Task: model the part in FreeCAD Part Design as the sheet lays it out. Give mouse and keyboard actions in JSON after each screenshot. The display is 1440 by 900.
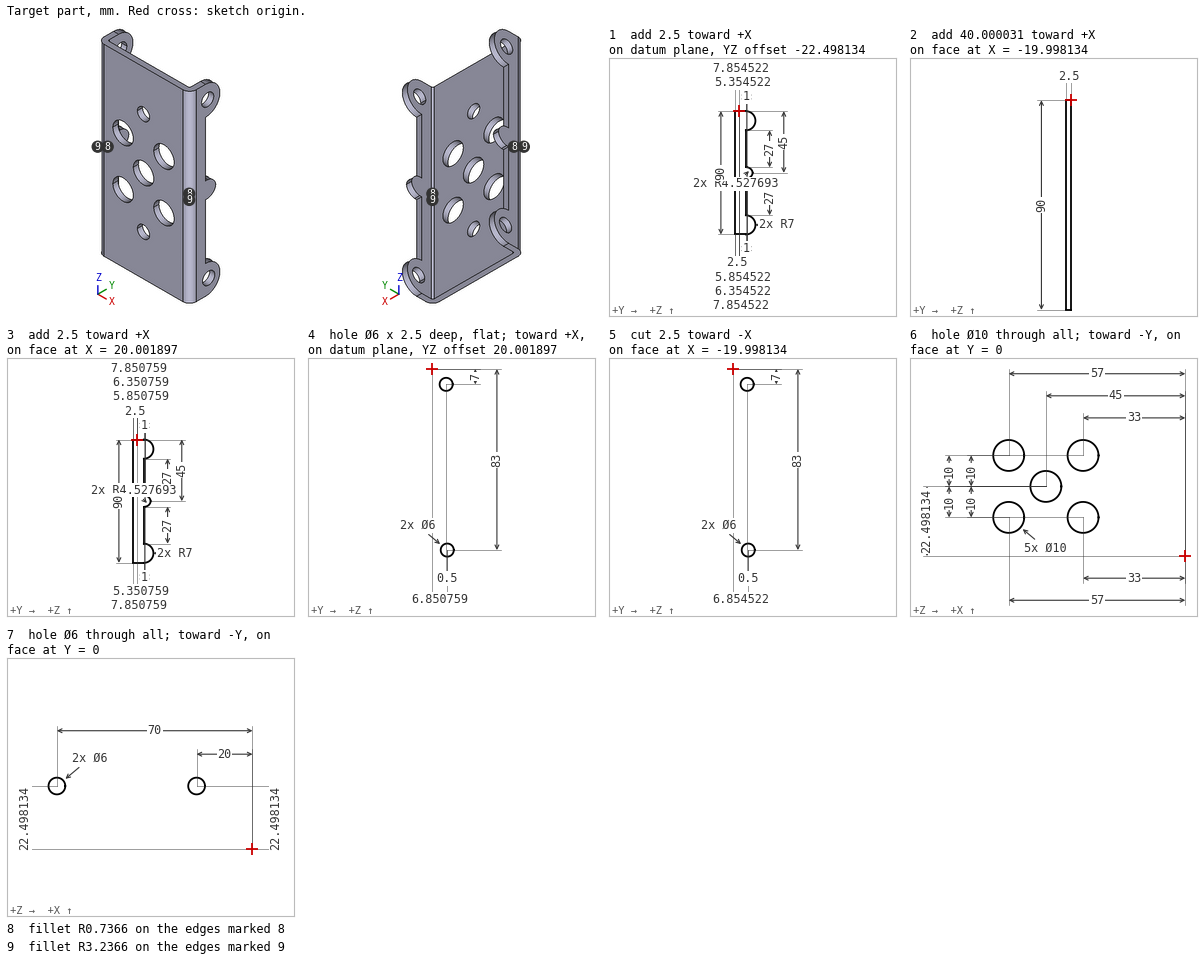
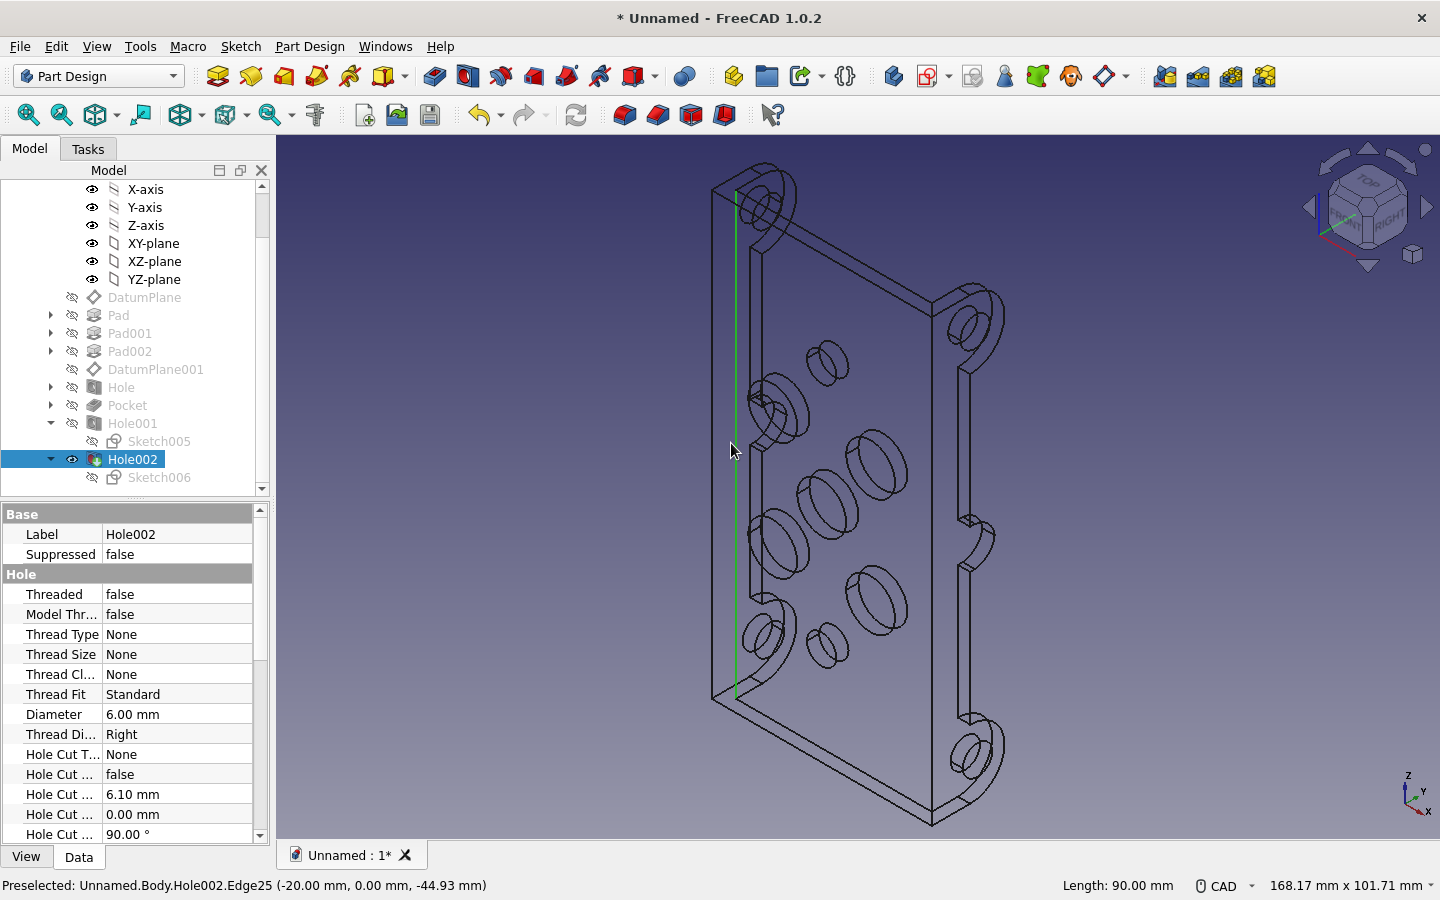
{"action": "scroll", "coordinate": [932, 556], "scroll_direction": "up", "scroll_amount": 6}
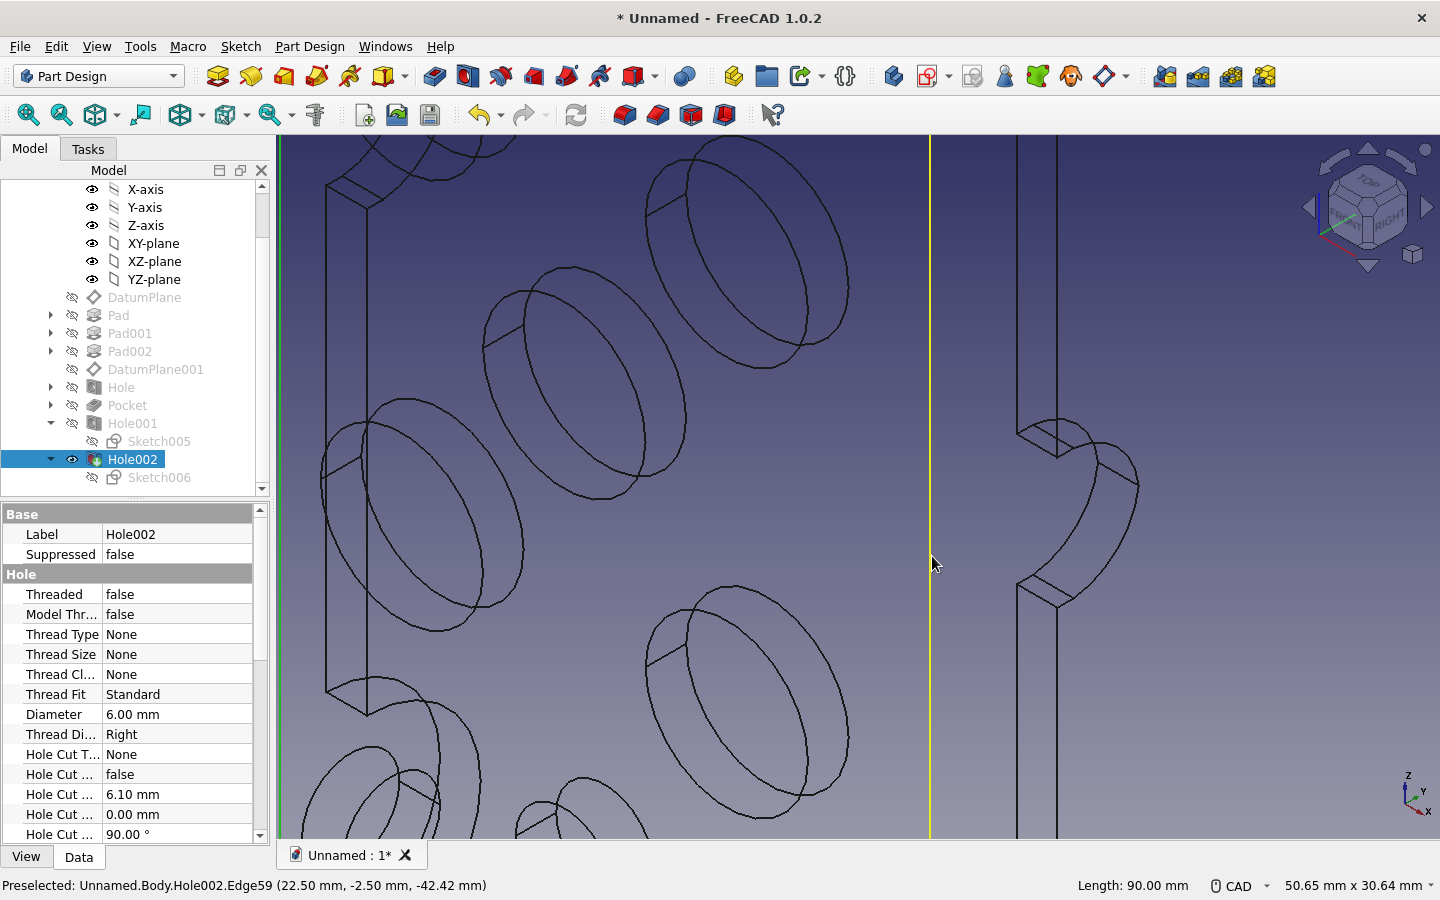
{"action": "left_click", "coordinate": [29, 116]}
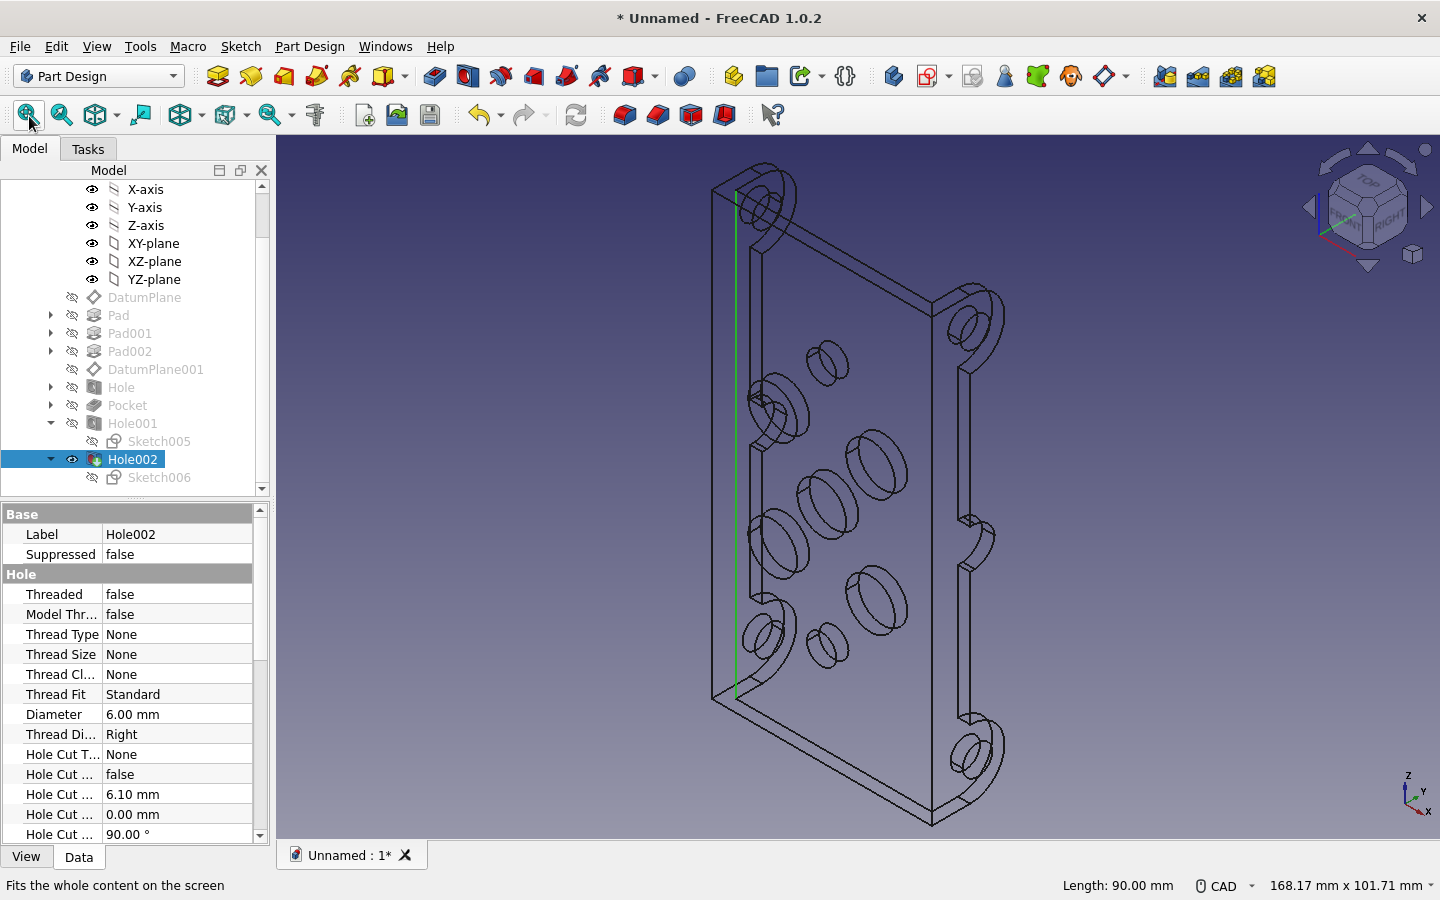
{"action": "key", "text": "2"}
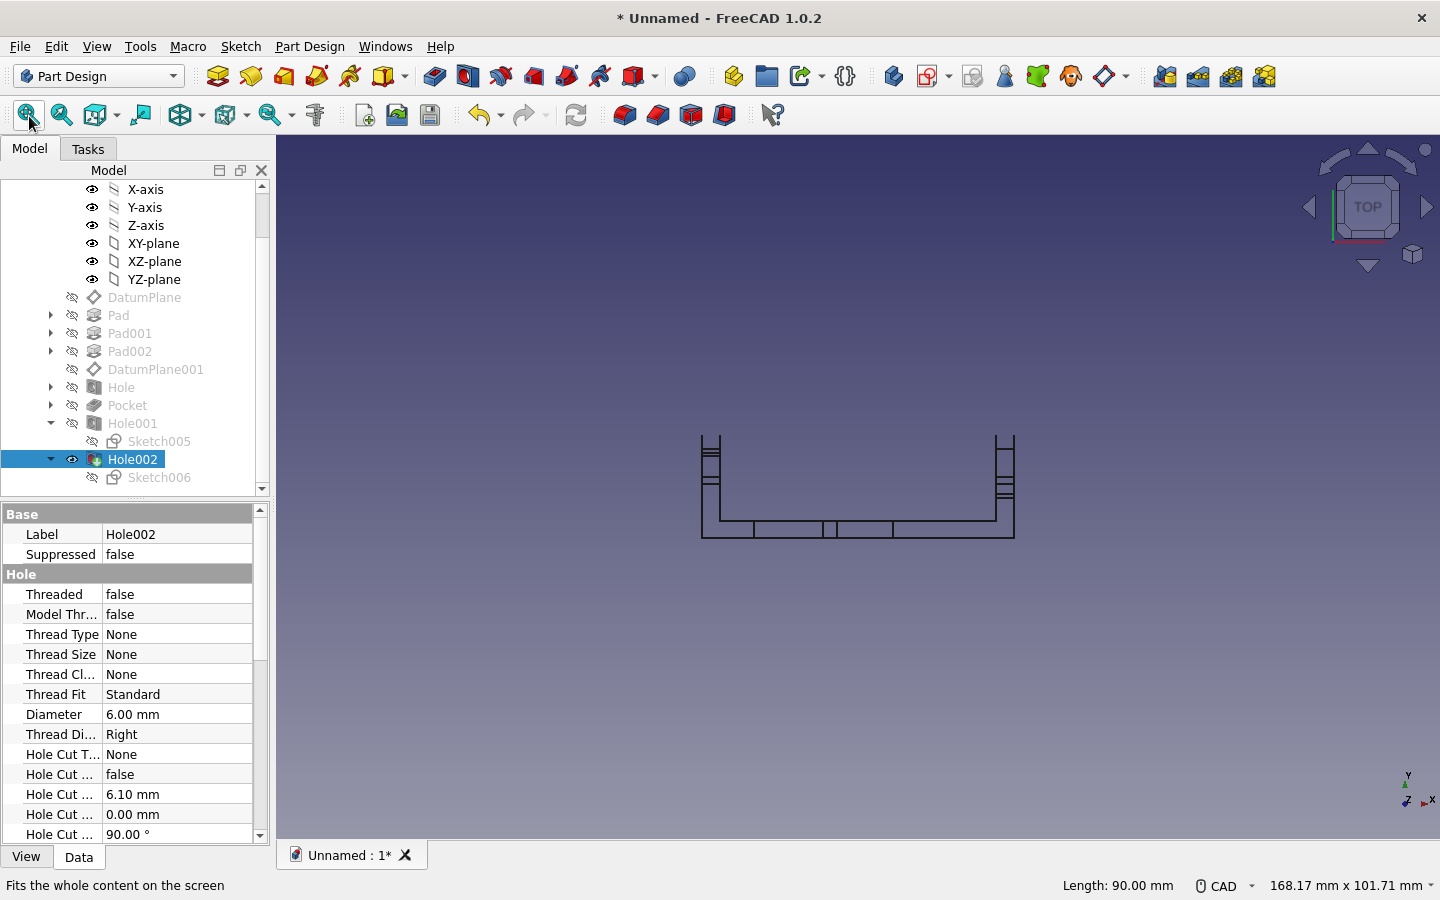
{"action": "left_click", "coordinate": [29, 116]}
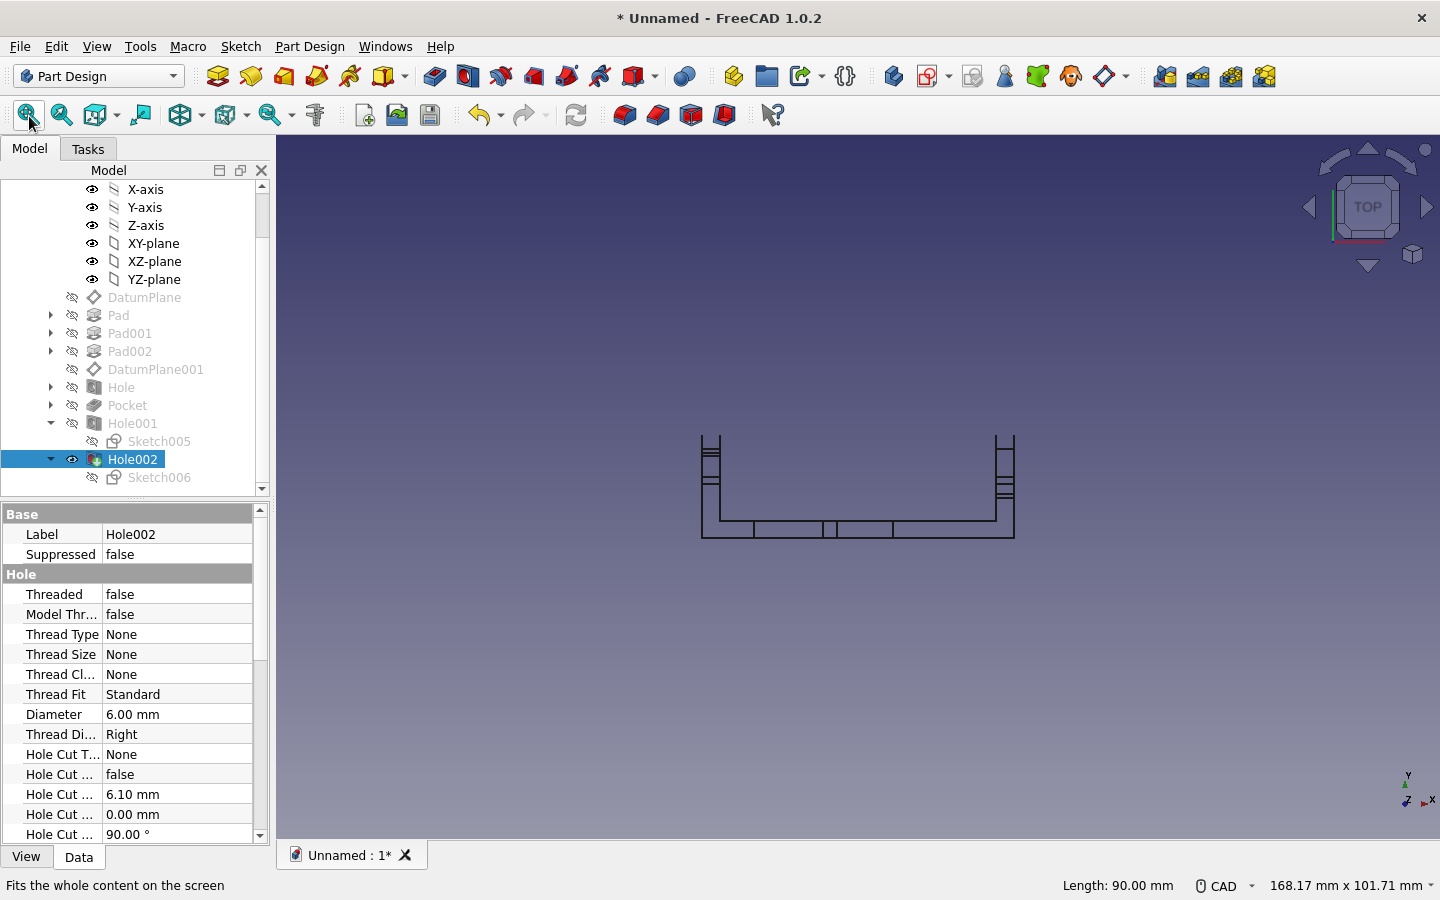
{"action": "scroll", "coordinate": [996, 520], "scroll_direction": "up", "scroll_amount": 6}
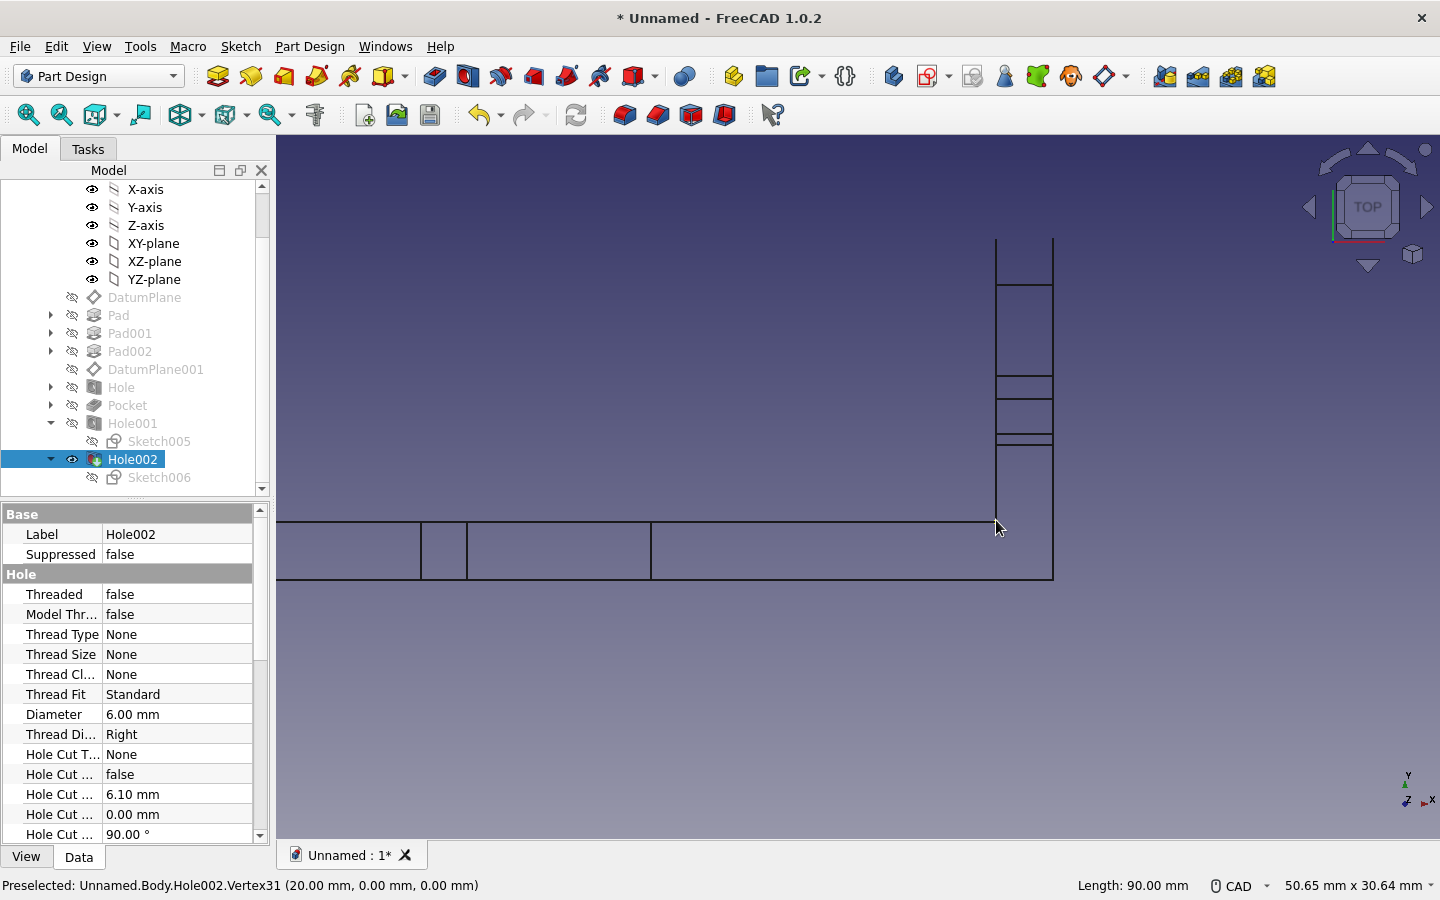
{"action": "left_click", "coordinate": [29, 116]}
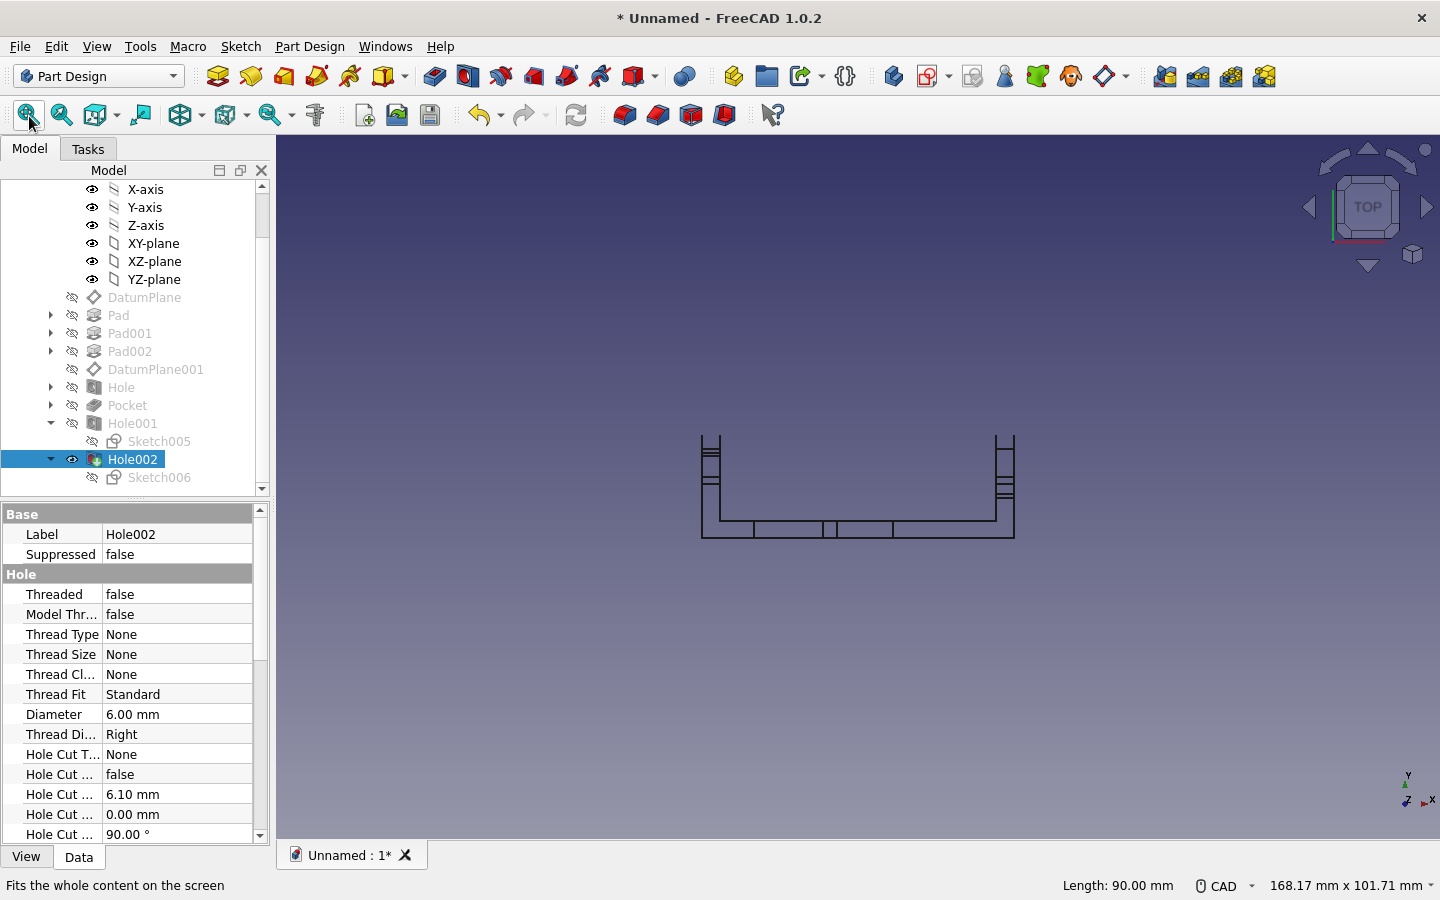
{"action": "key", "text": "1"}